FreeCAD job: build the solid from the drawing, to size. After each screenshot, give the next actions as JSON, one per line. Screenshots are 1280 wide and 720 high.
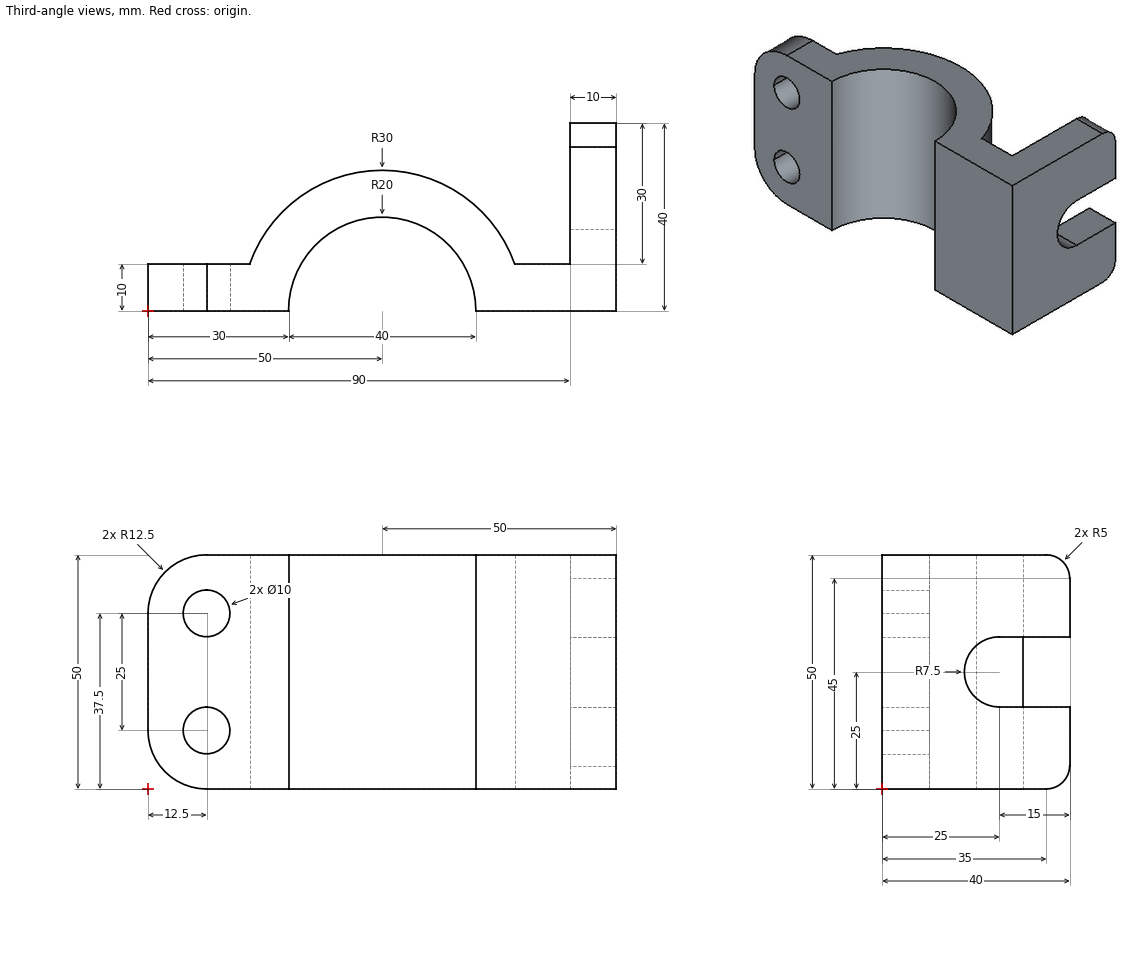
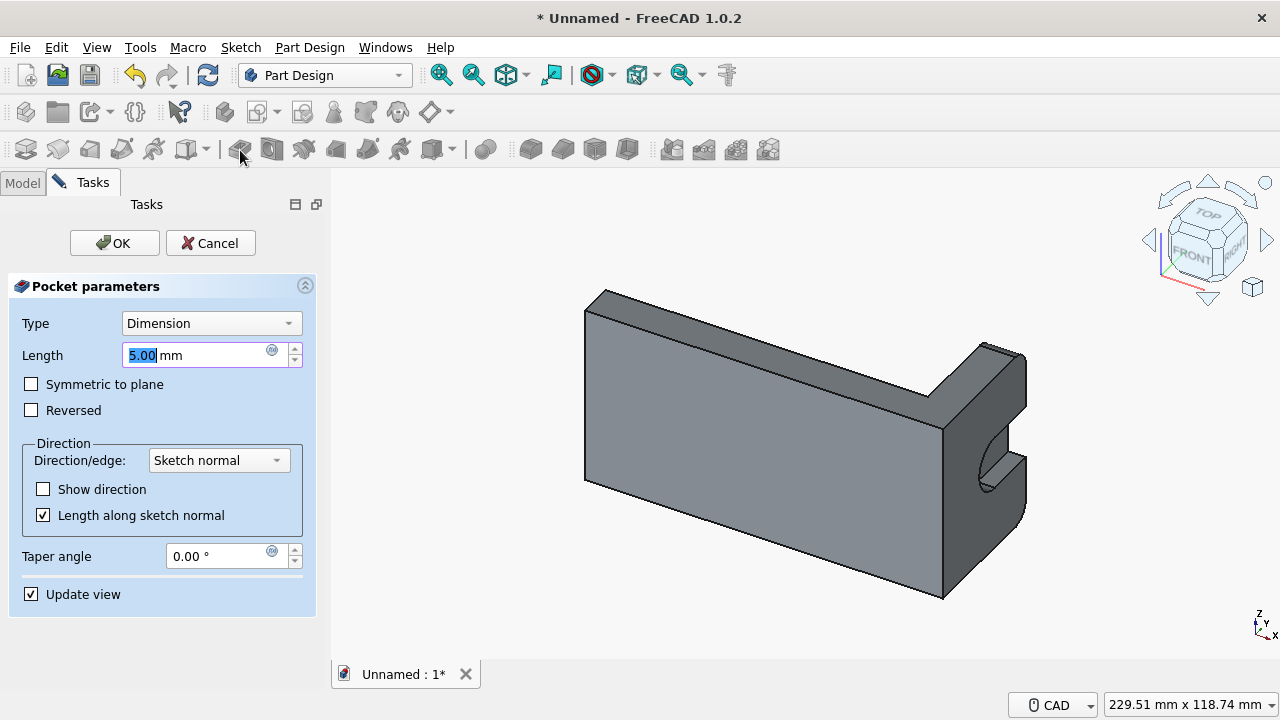
{"action": "type", "text": "50"}
{"action": "key", "text": "Tab"}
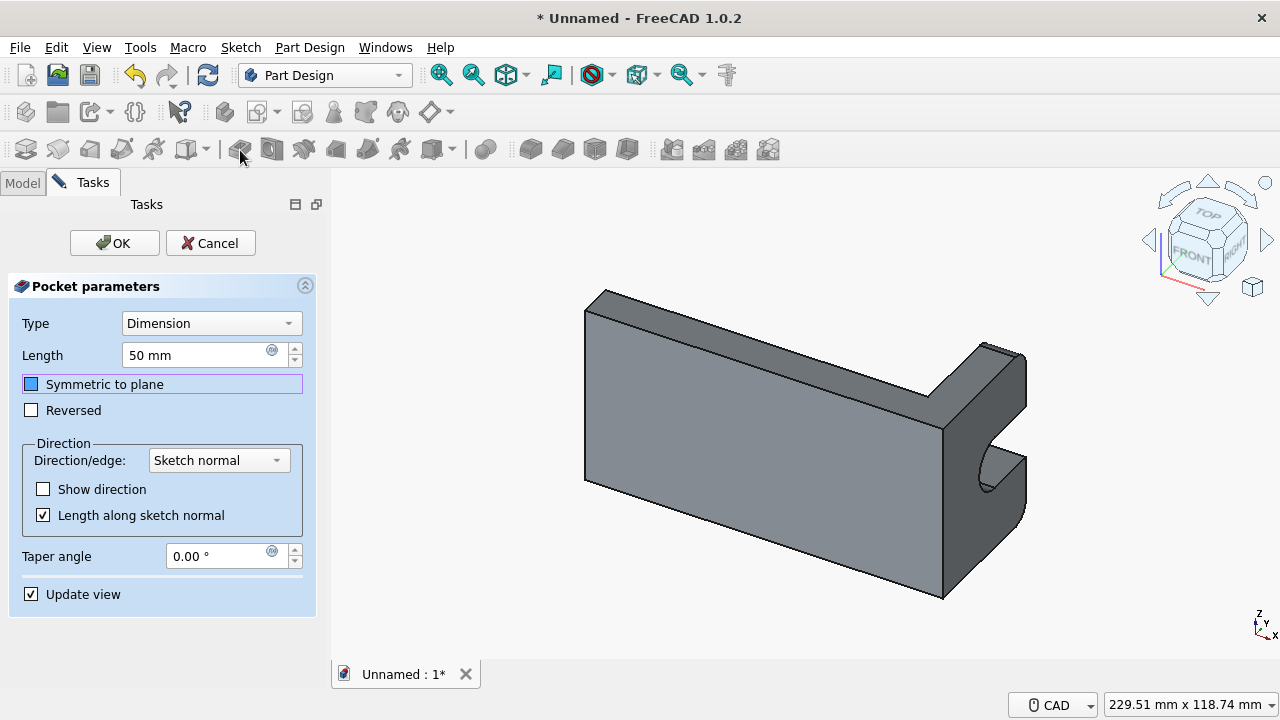
{"action": "left_click", "coordinate": [115, 243]}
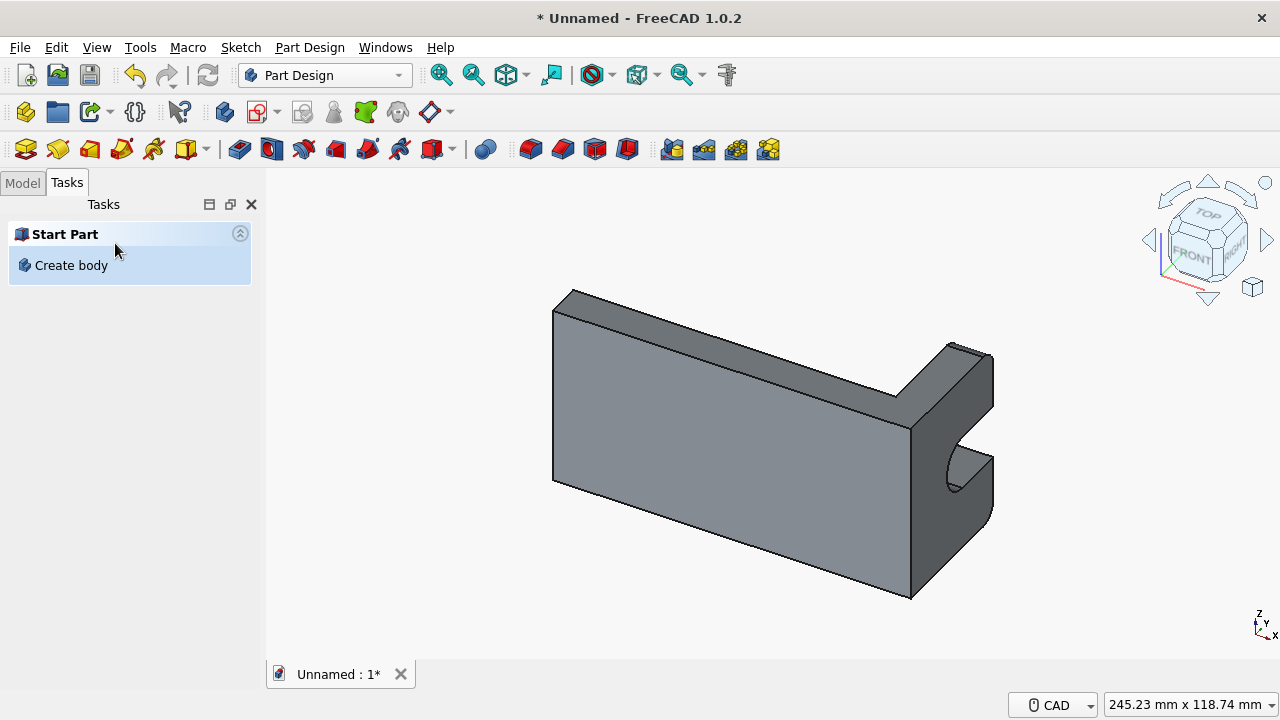
{"action": "key", "text": "4"}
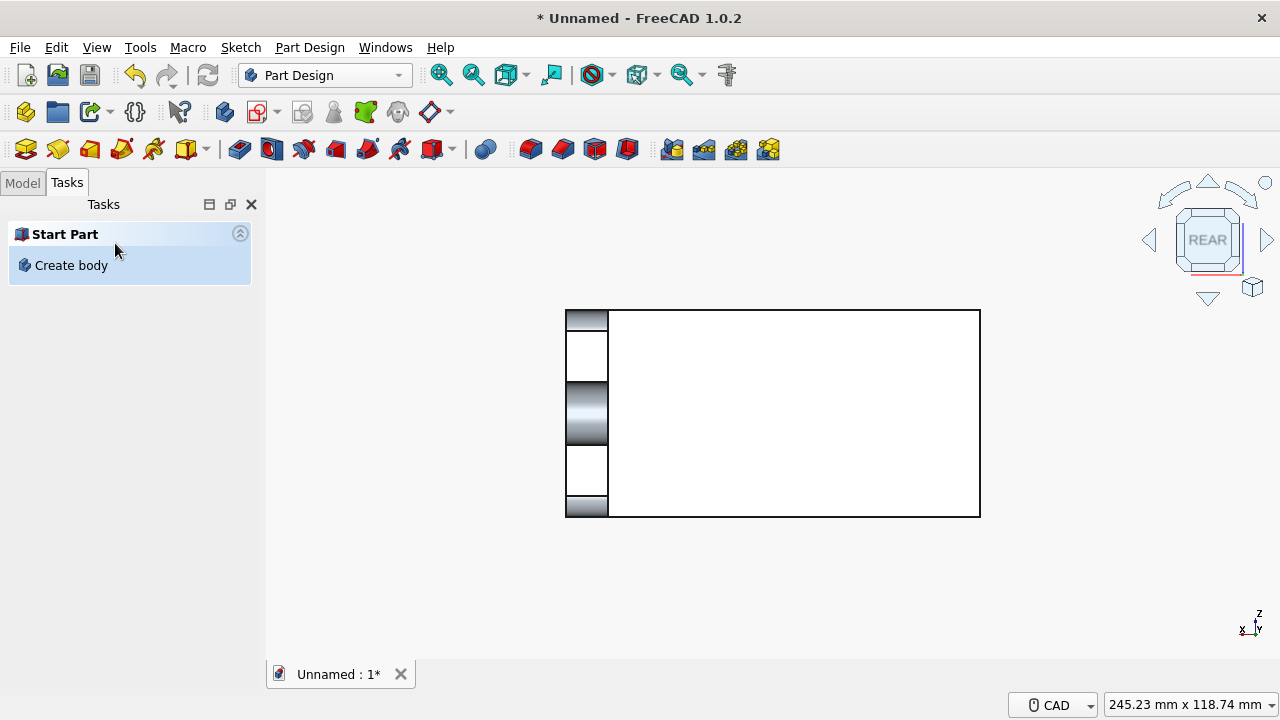
{"action": "left_click", "coordinate": [442, 76]}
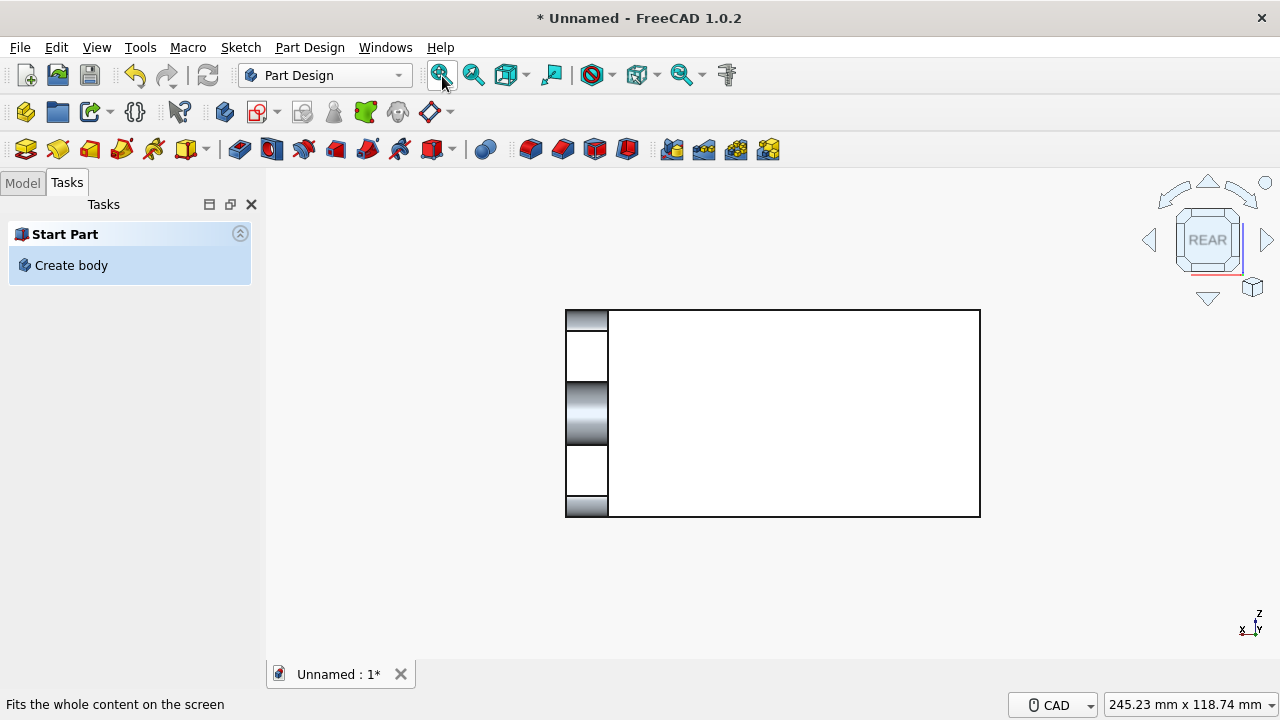
{"action": "left_click", "coordinate": [741, 413]}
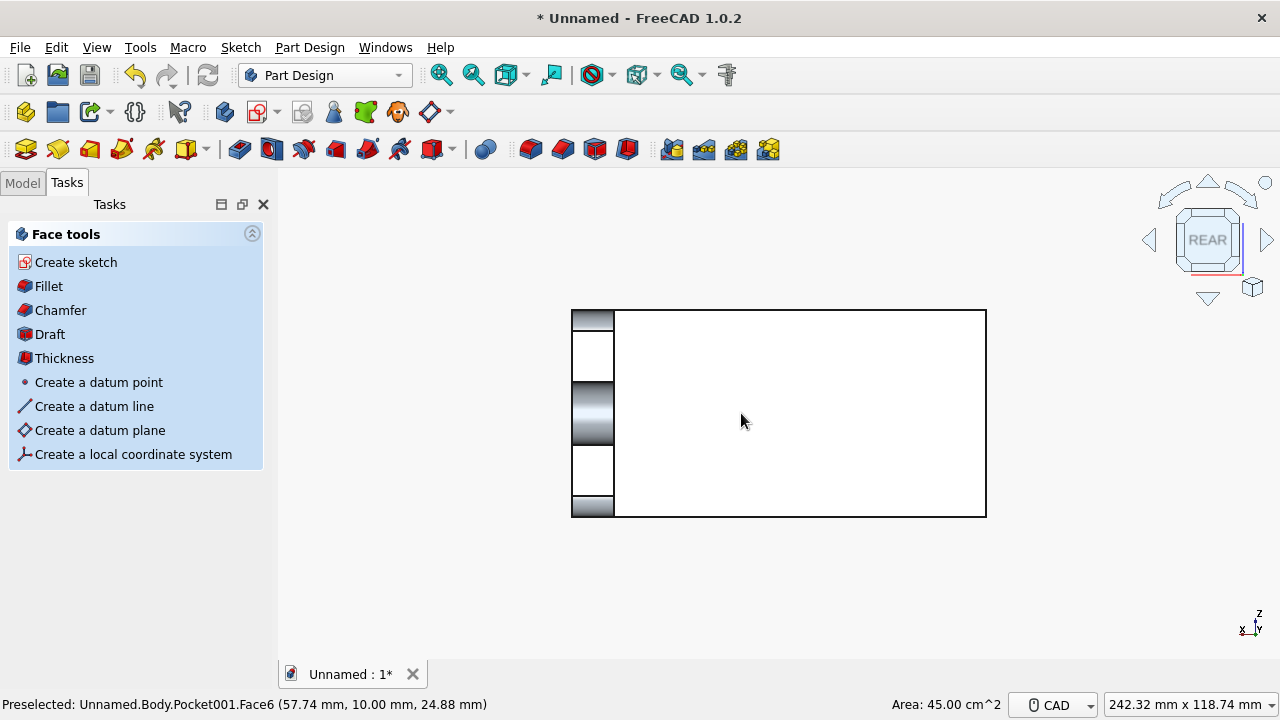
{"action": "left_click", "coordinate": [258, 112]}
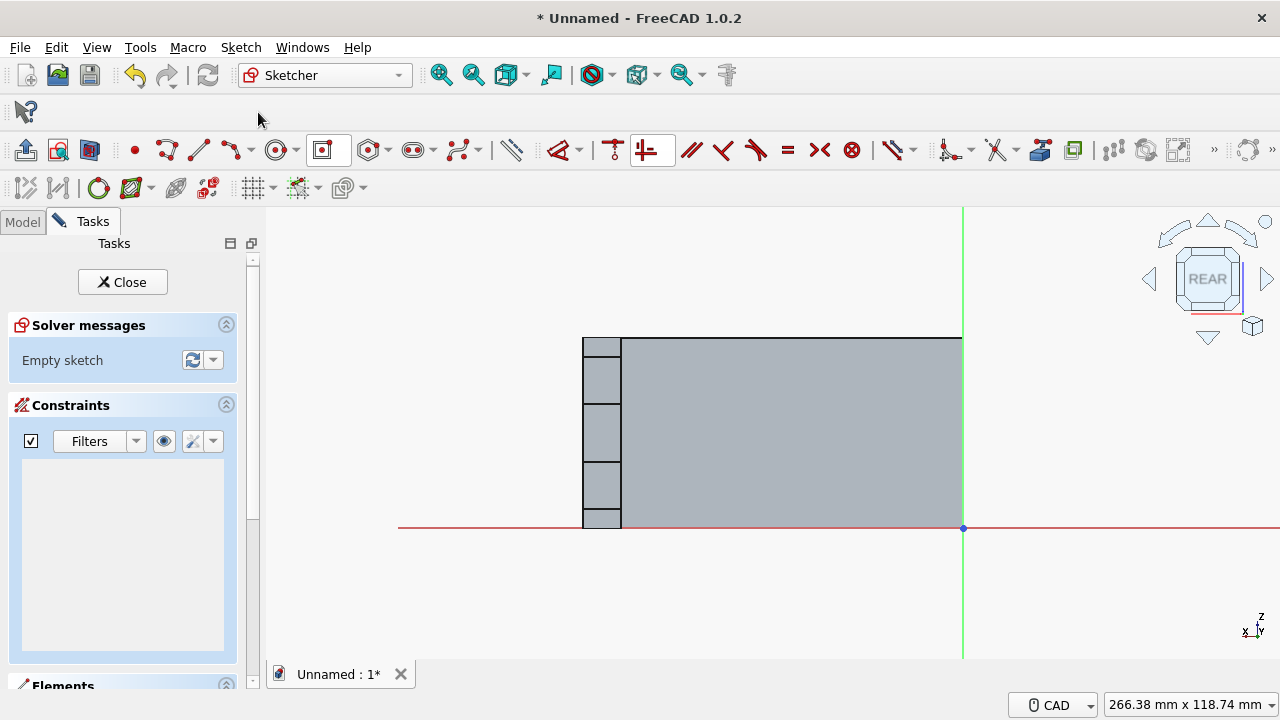
{"action": "left_click", "coordinate": [90, 150]}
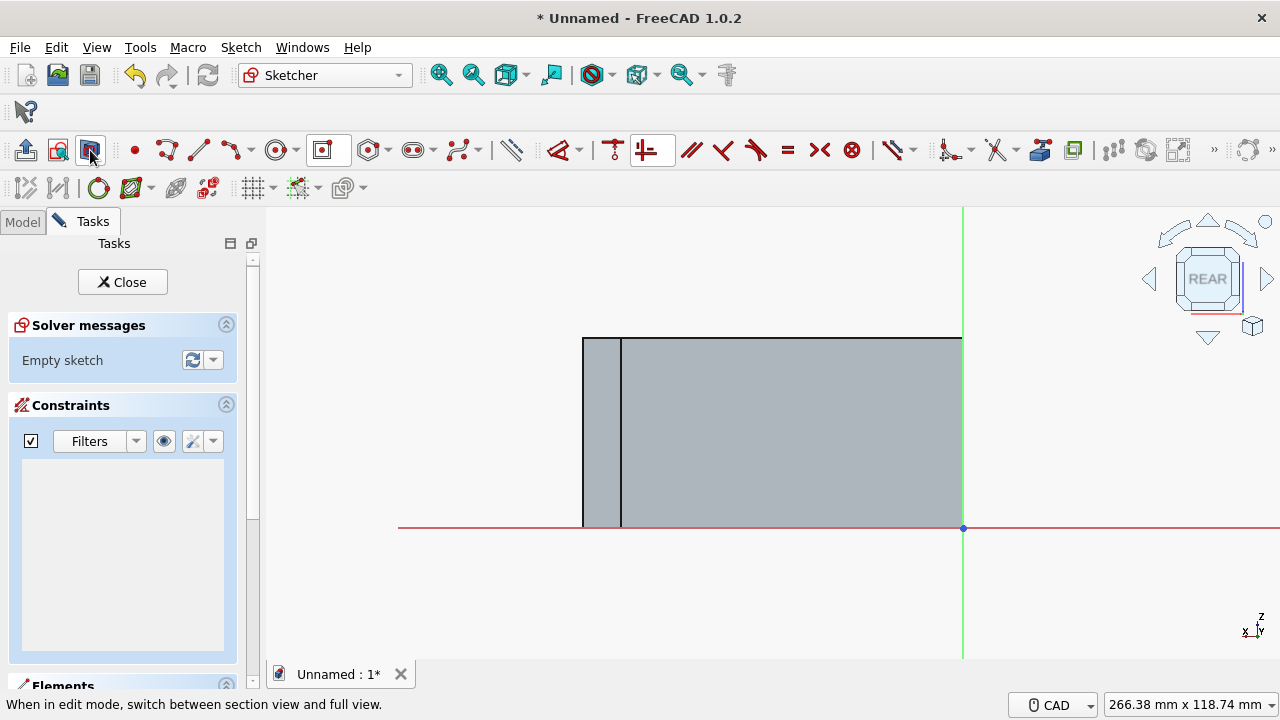
{"action": "scroll", "coordinate": [1115, 433], "scroll_direction": "up", "scroll_amount": 2}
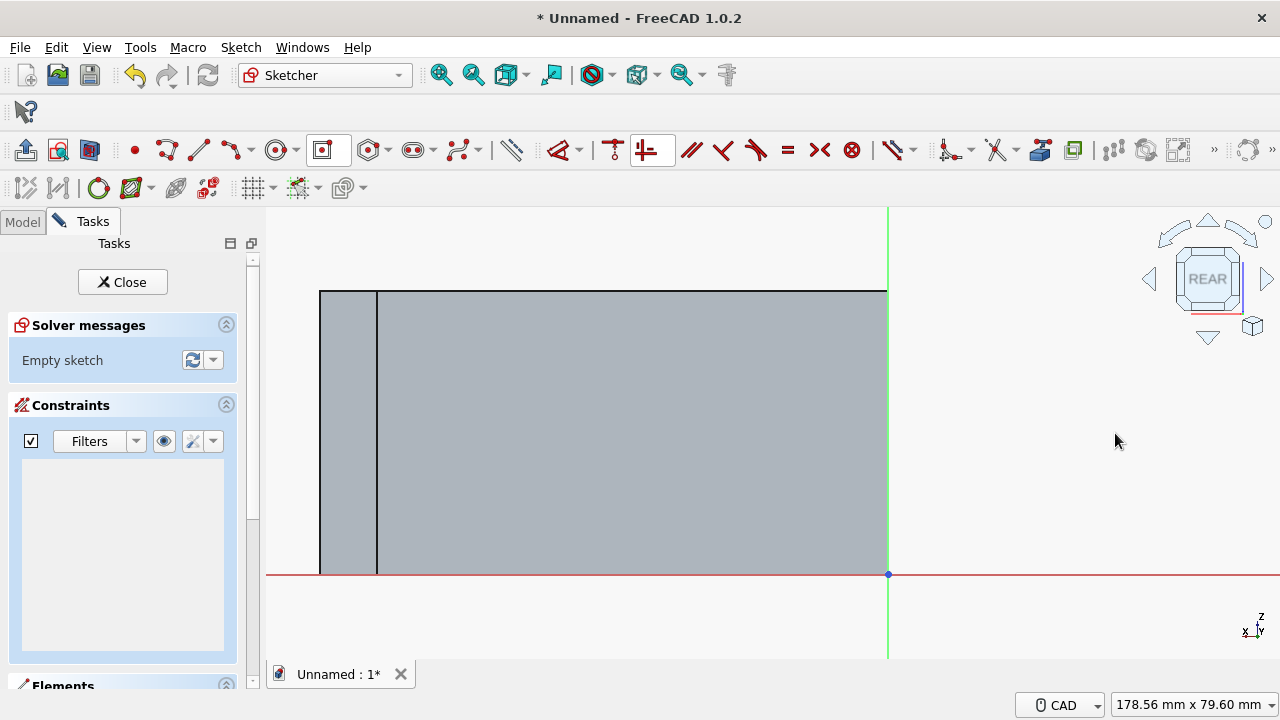
{"action": "left_click", "coordinate": [168, 150]}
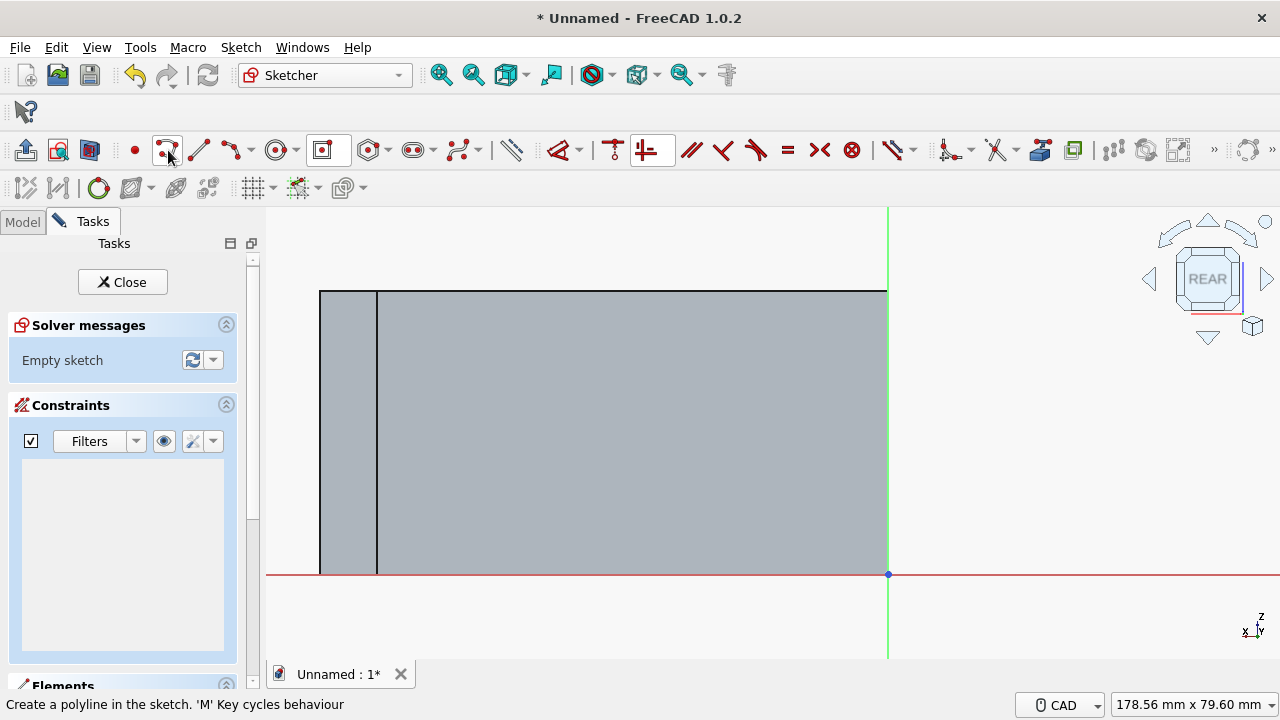
{"action": "left_click", "coordinate": [888, 362]}
{"action": "left_click", "coordinate": [879, 291]}
{"action": "left_click", "coordinate": [817, 291]}
{"action": "right_click", "coordinate": [817, 291]}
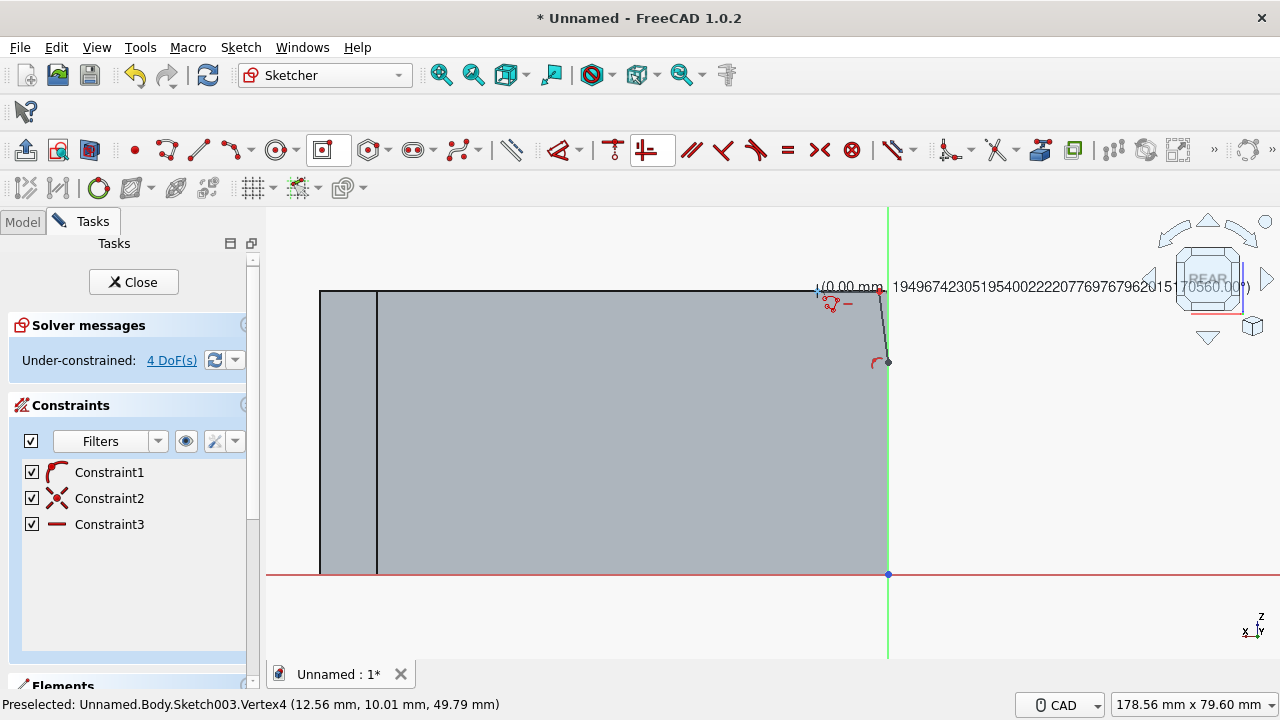
{"action": "left_click", "coordinate": [232, 150]}